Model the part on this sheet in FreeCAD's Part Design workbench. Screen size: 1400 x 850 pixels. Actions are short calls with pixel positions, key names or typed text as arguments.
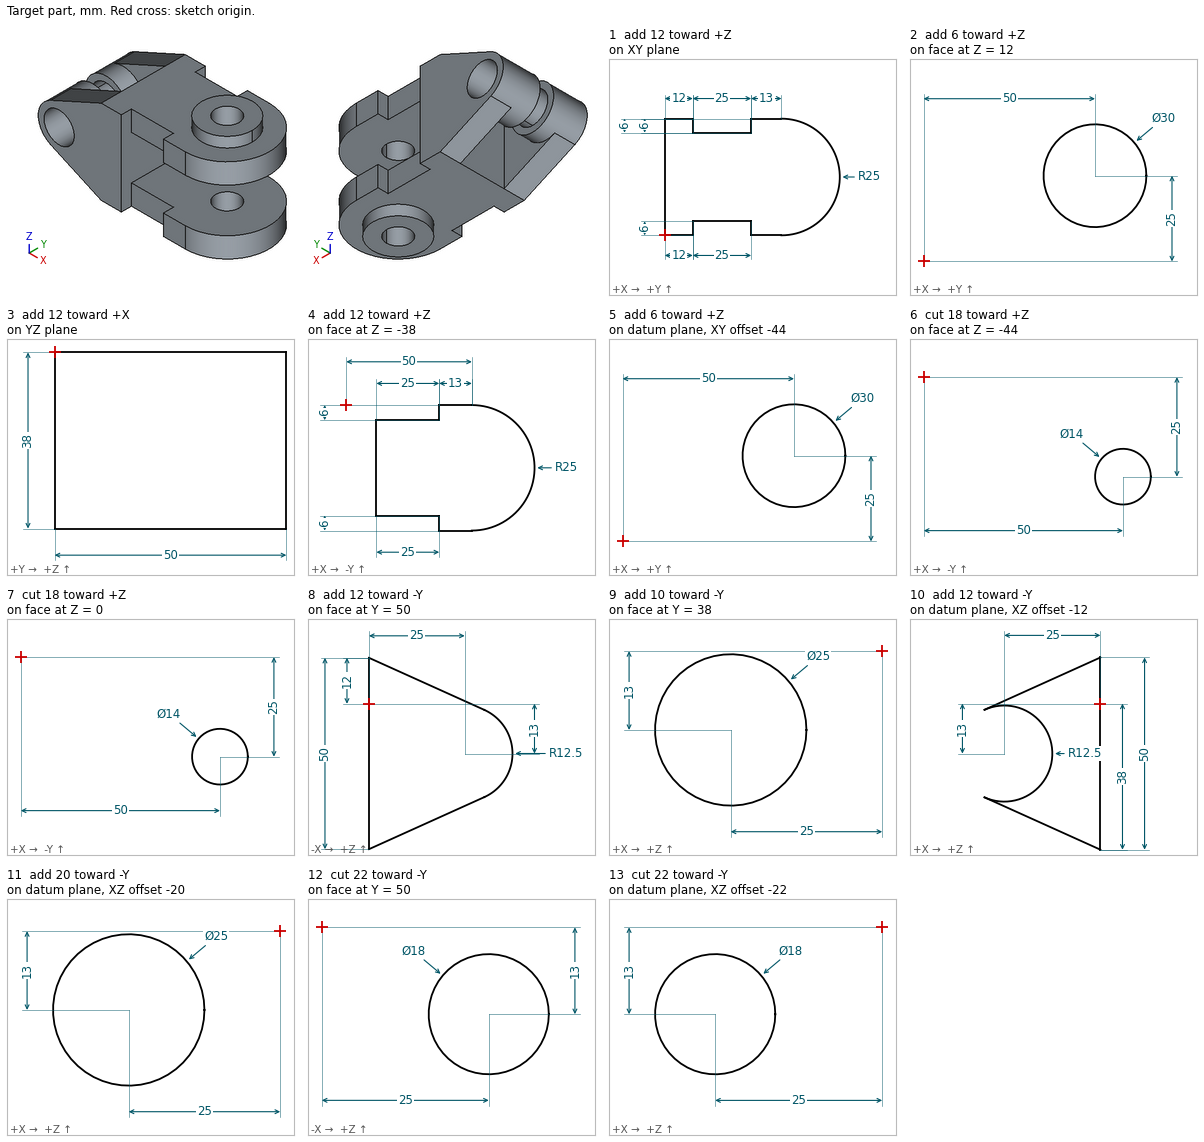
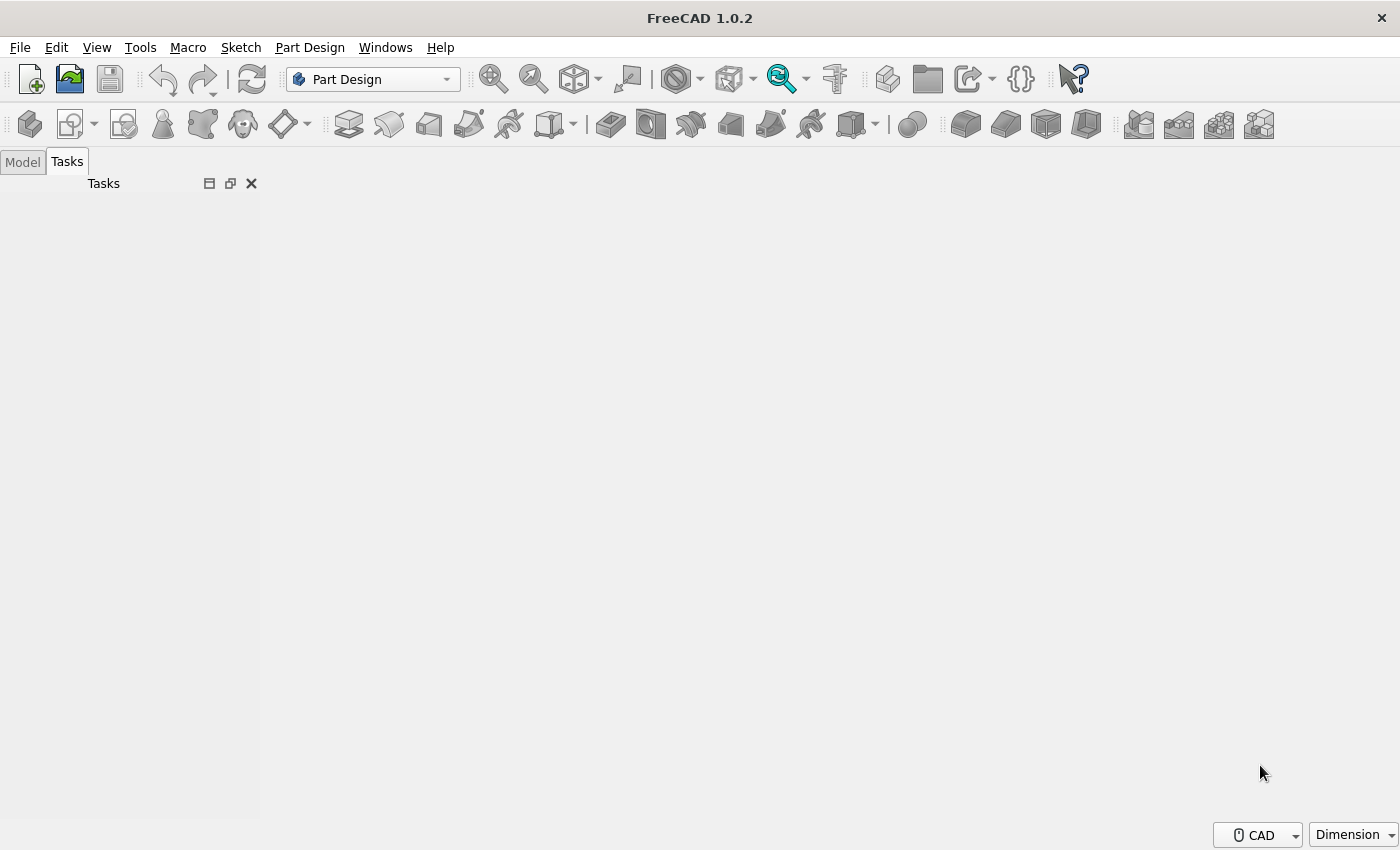
click(30, 80)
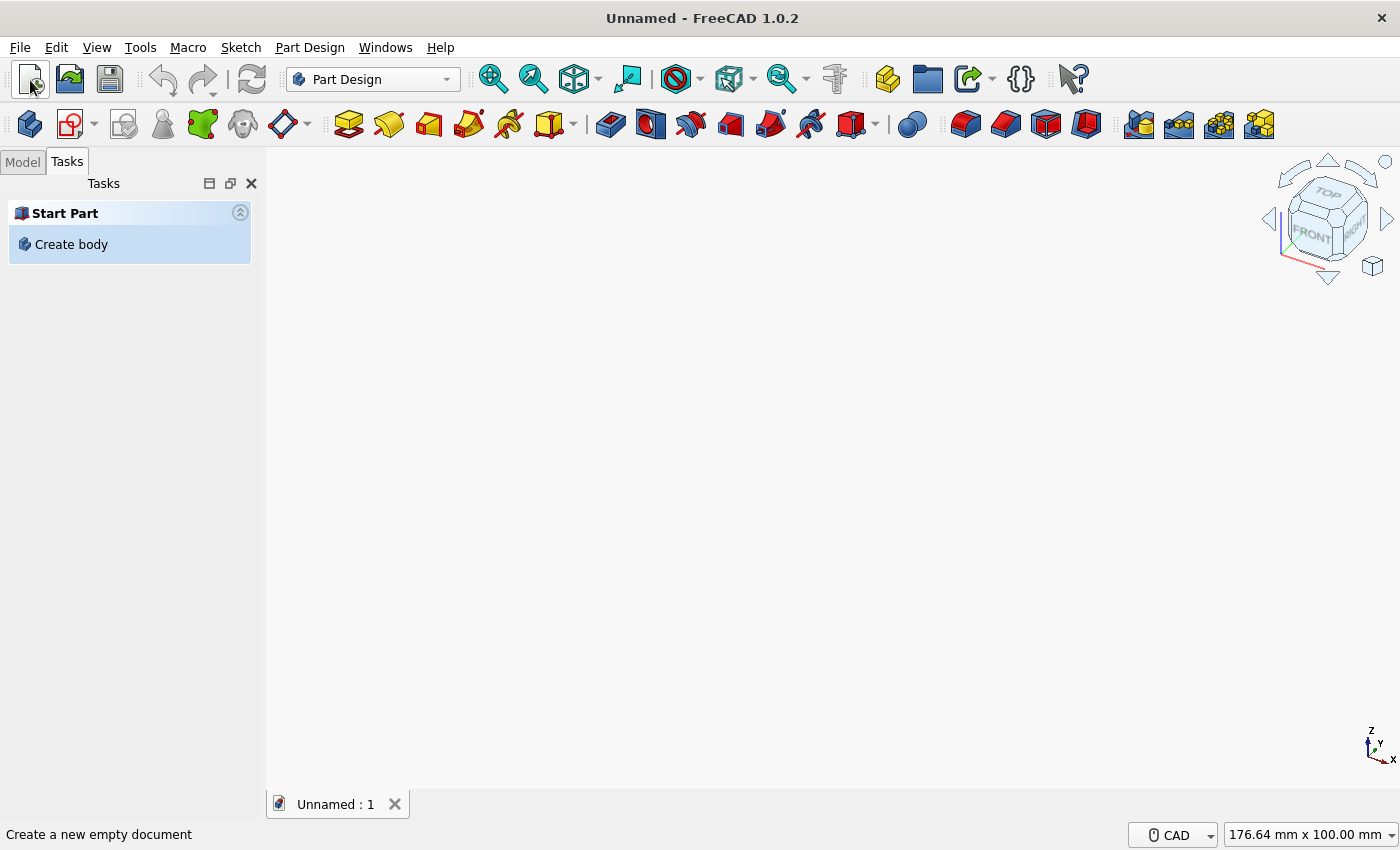
click(70, 124)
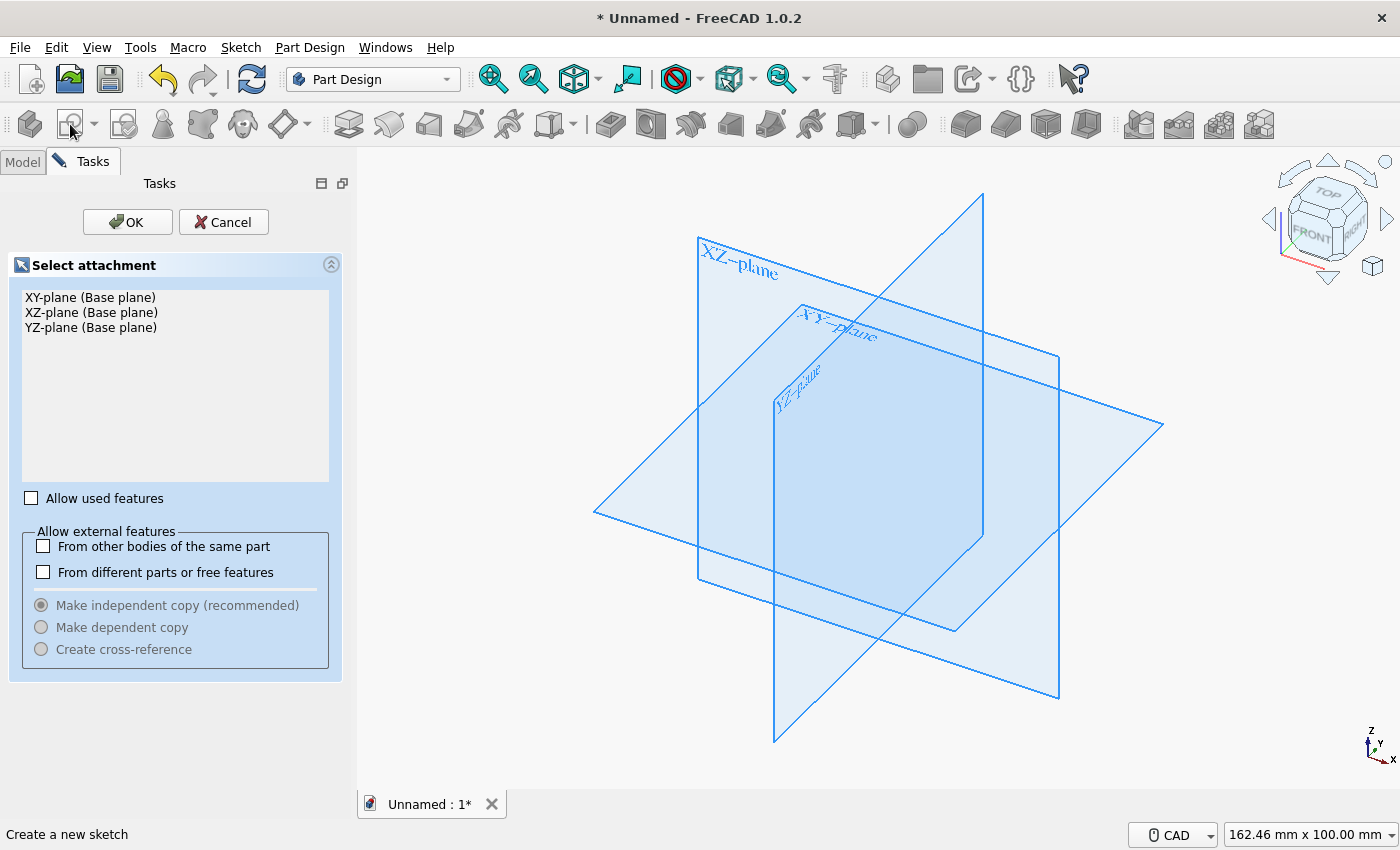
click(82, 298)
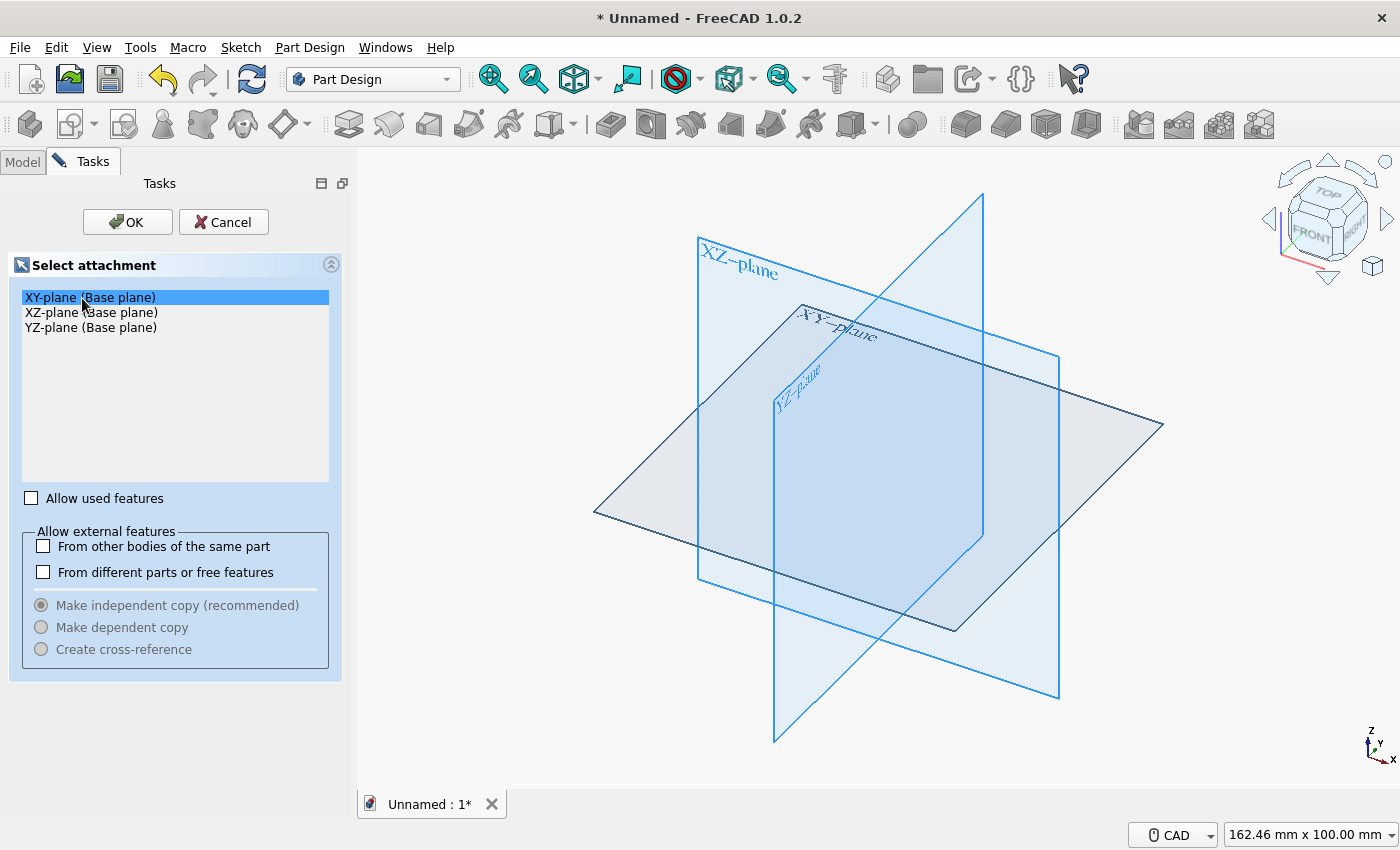
click(128, 222)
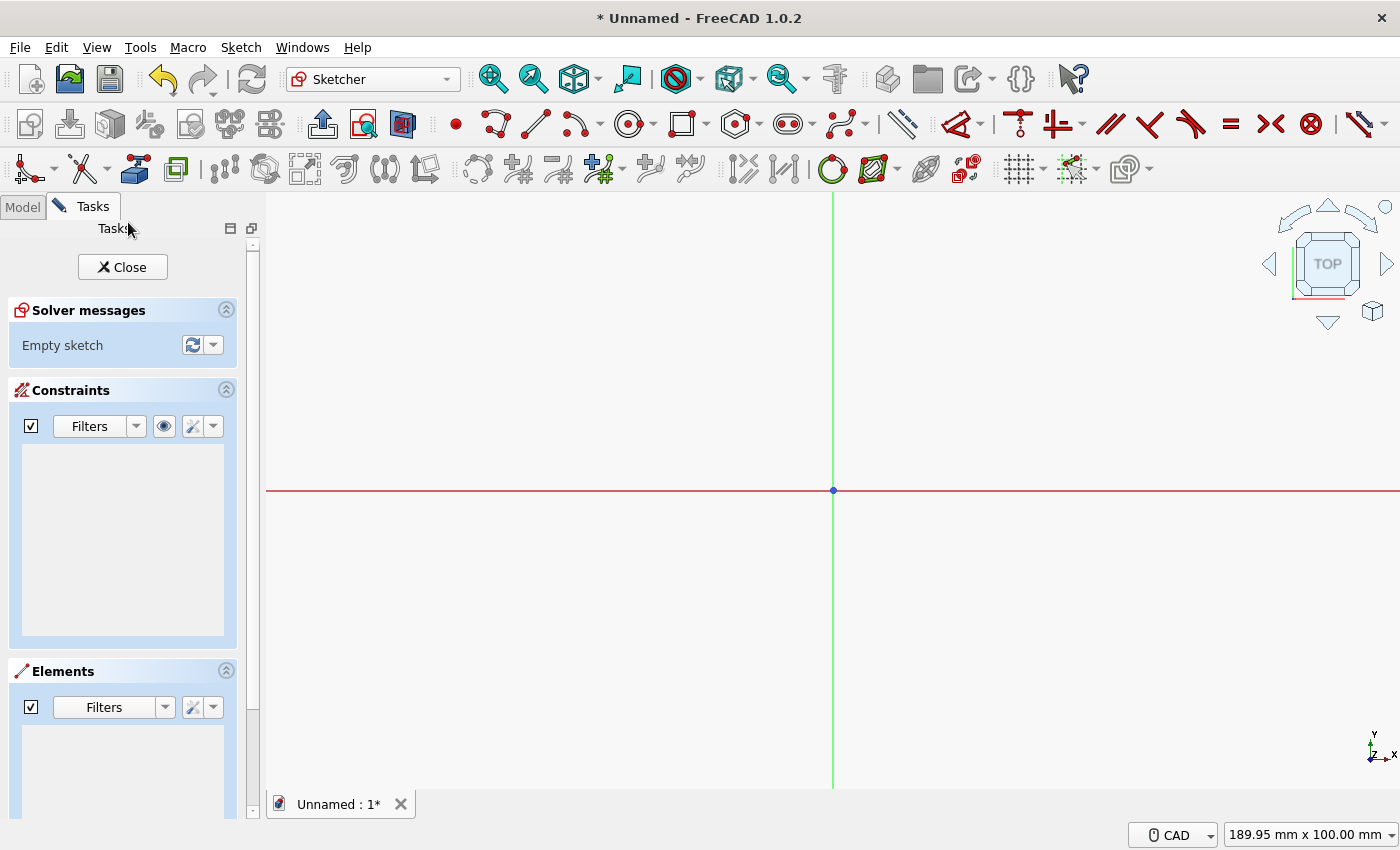
scroll(294, 761, down, 1)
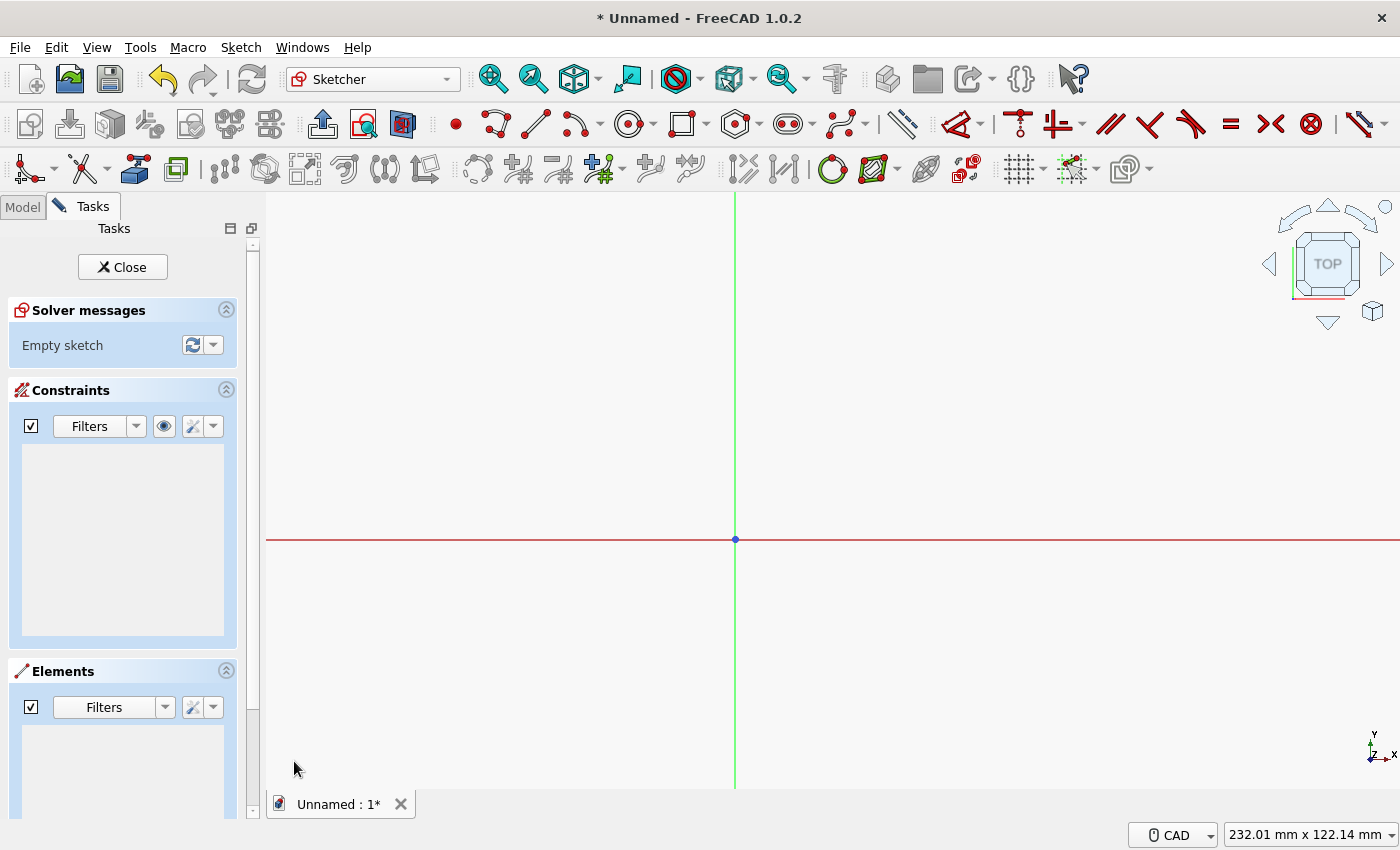
scroll(1232, 269, up, 2)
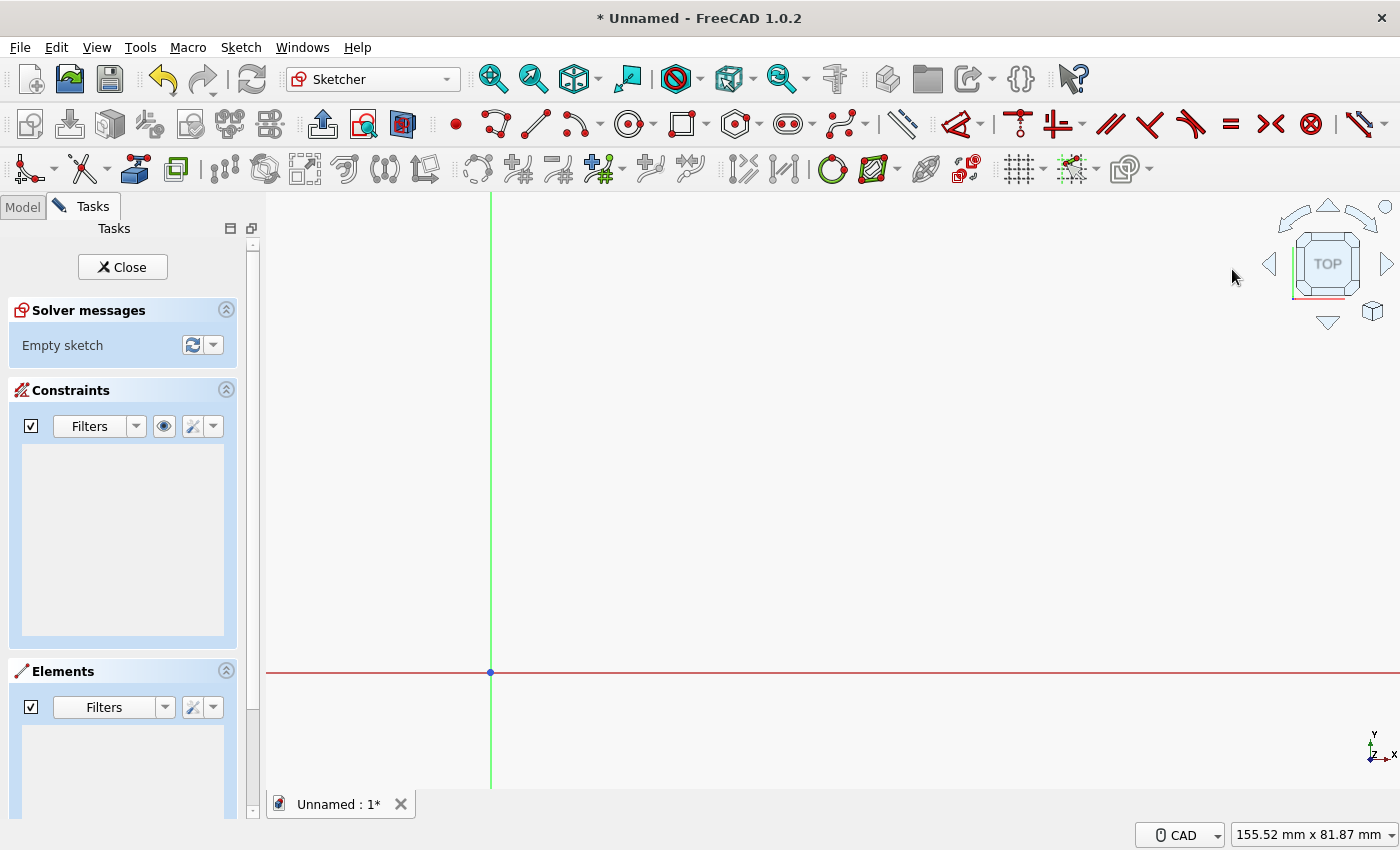
click(496, 124)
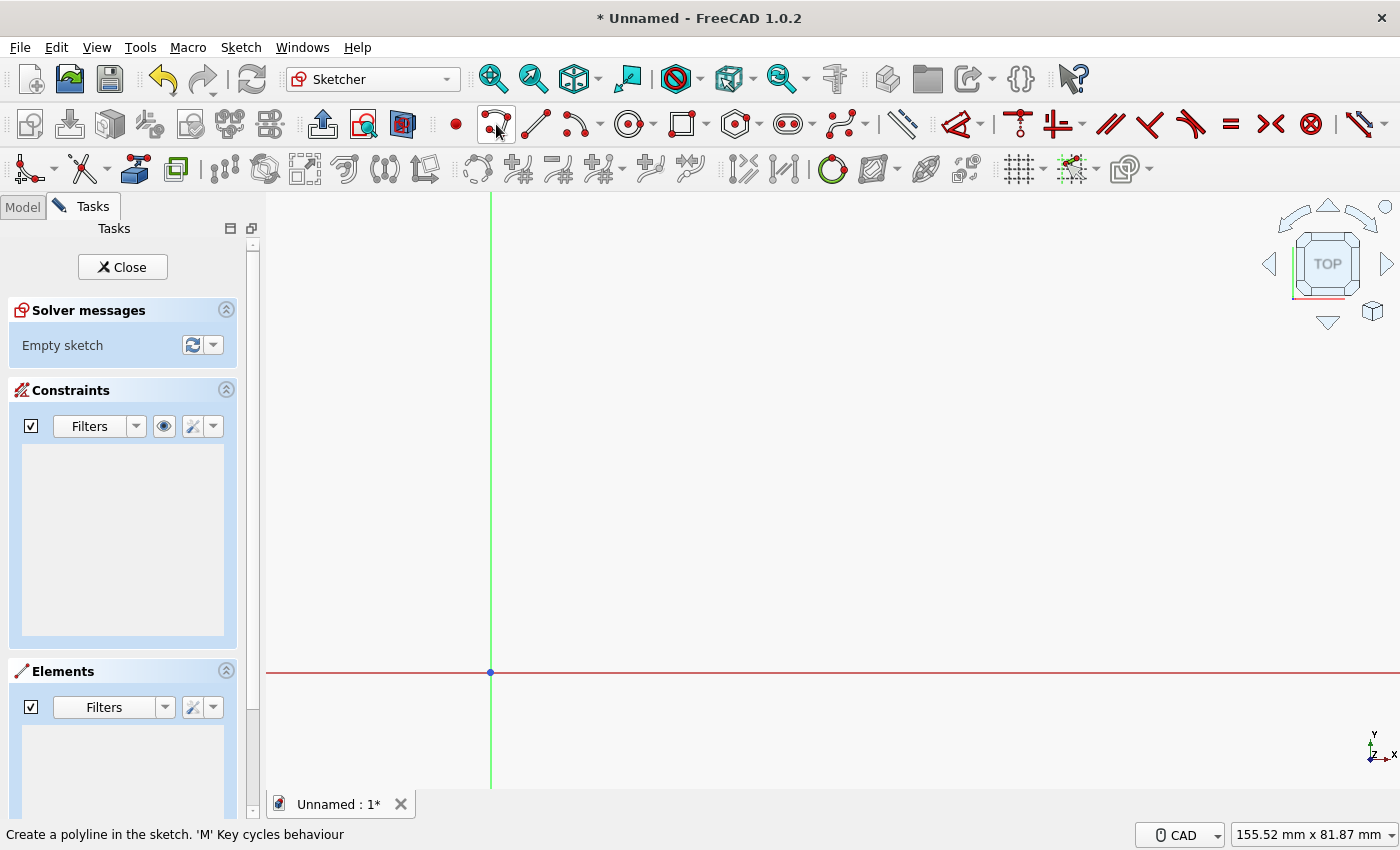
click(855, 308)
click(760, 308)
click(760, 352)
click(578, 352)
click(578, 308)
click(491, 308)
click(491, 673)
click(578, 664)
click(578, 629)
click(760, 629)
click(760, 673)
click(855, 664)
right_click(855, 664)